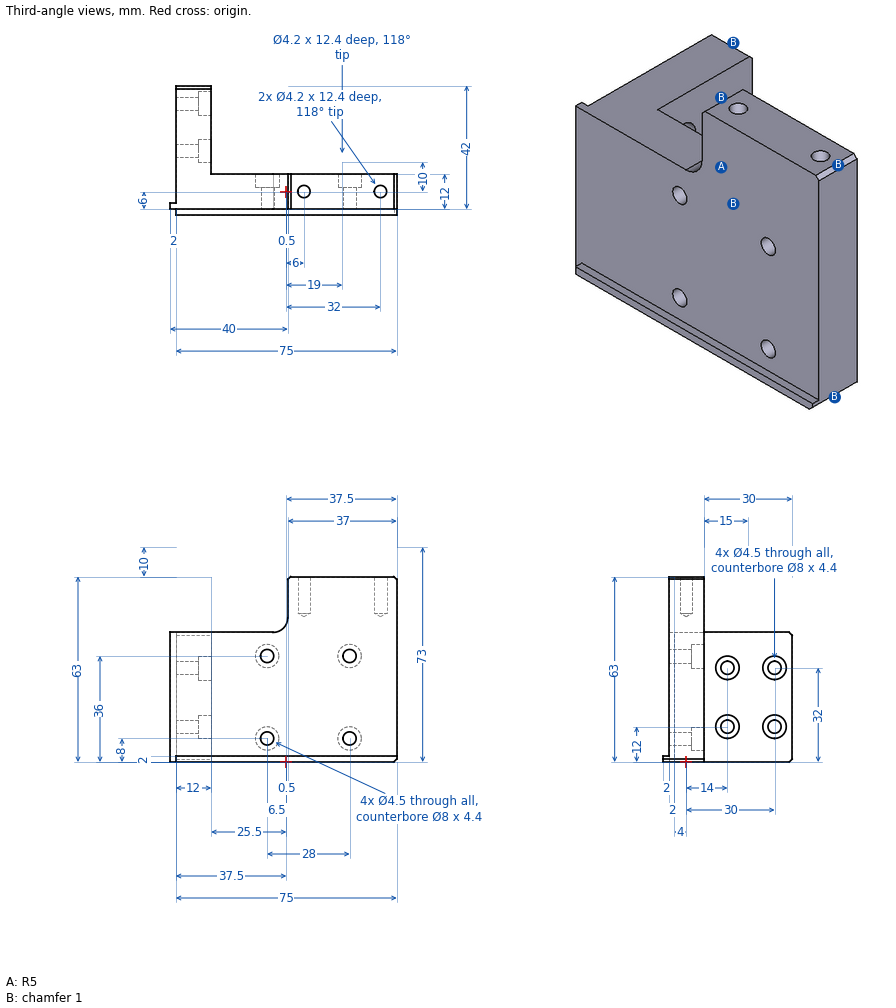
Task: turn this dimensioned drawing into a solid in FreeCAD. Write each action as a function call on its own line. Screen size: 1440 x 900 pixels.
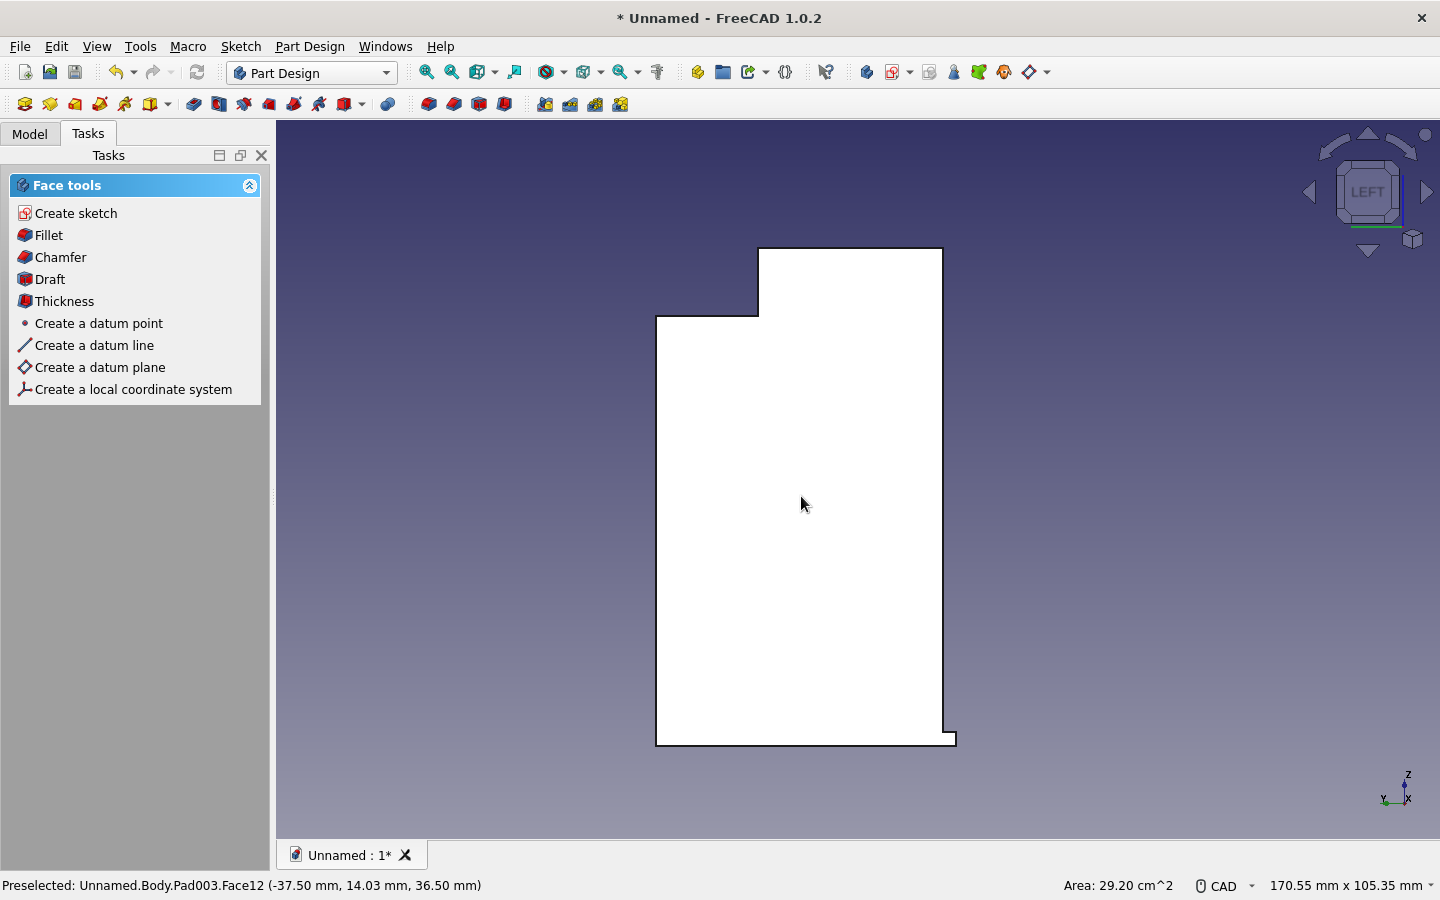
click(892, 72)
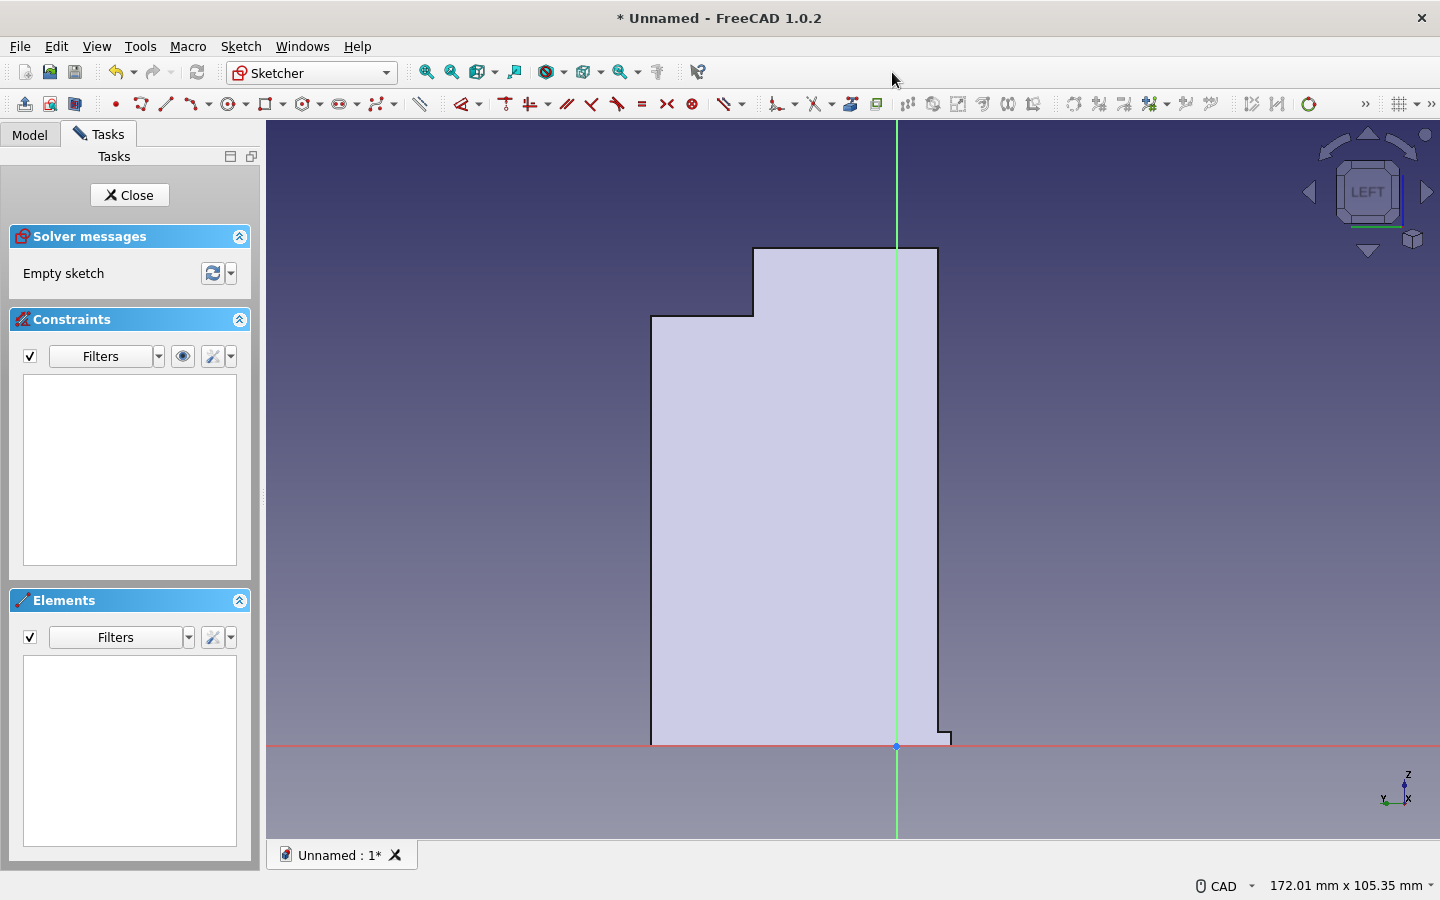
key(g)
key(r)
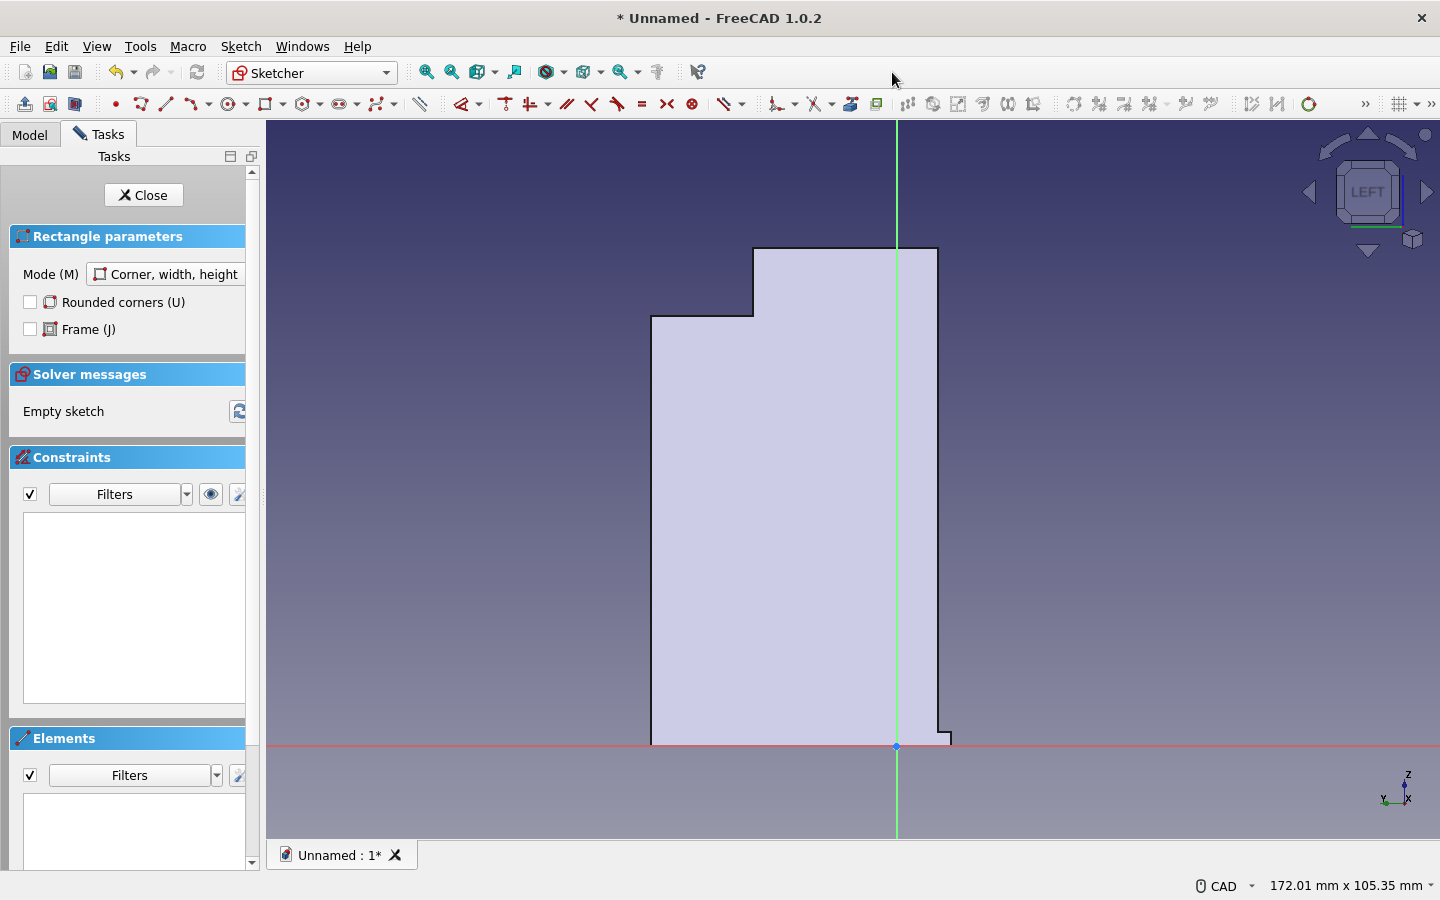
click(924, 316)
click(938, 746)
key(Escape)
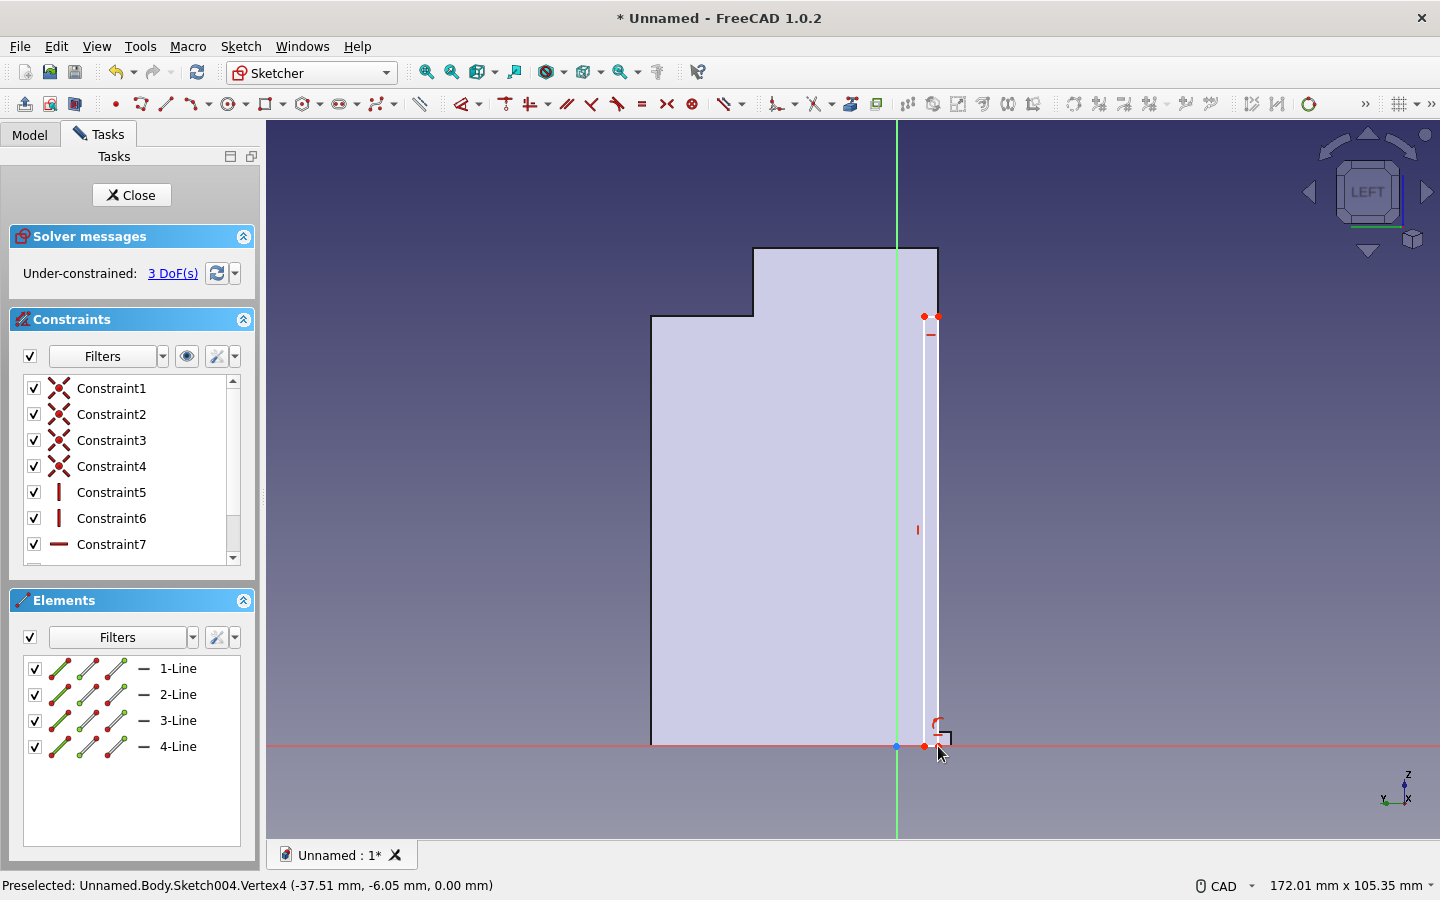
key(d)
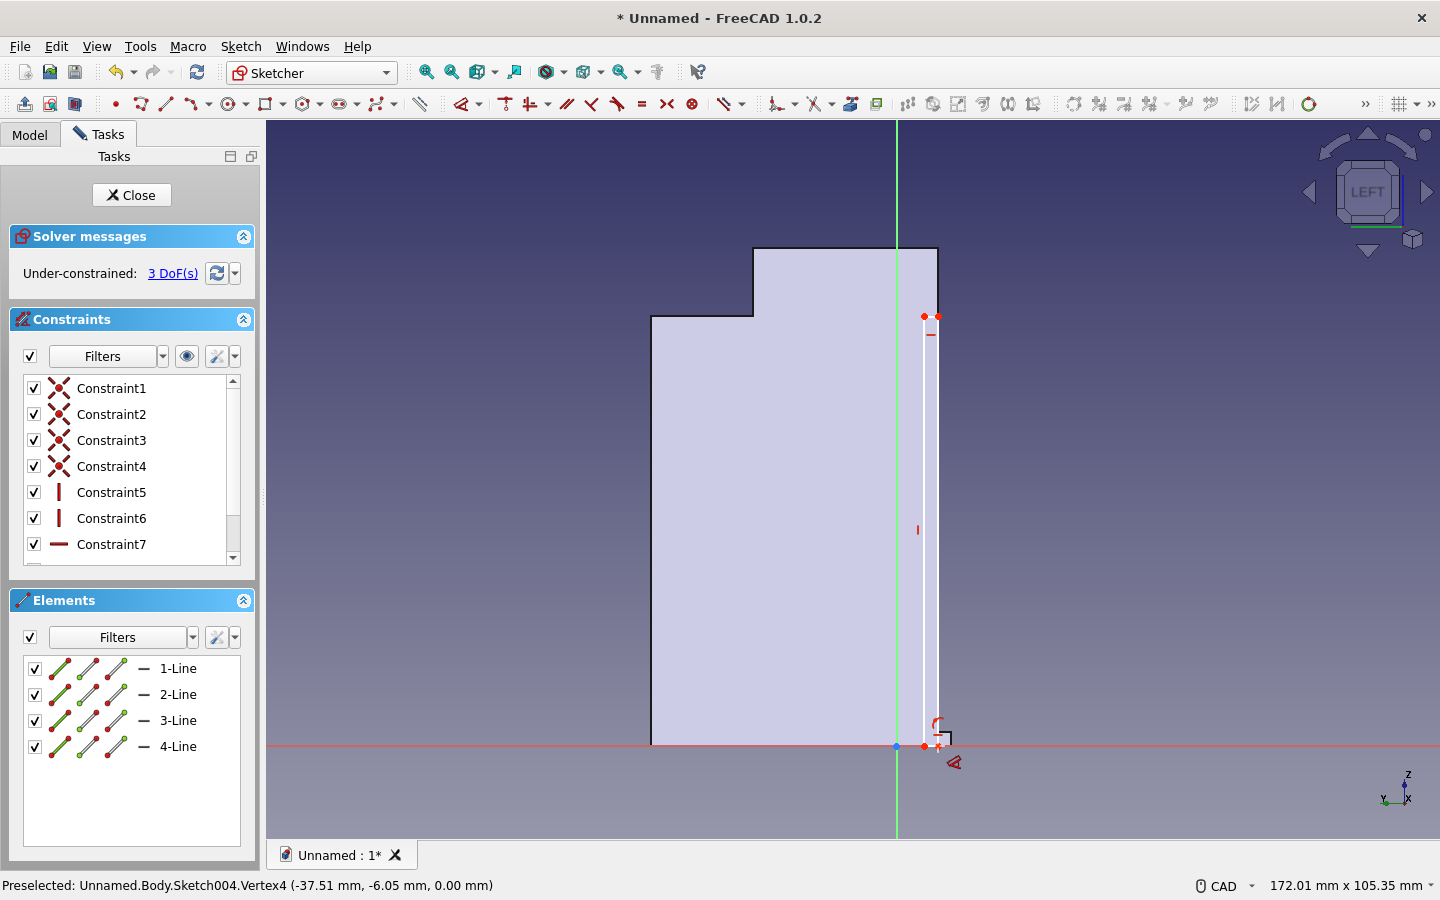
scroll(931, 746, up, 6)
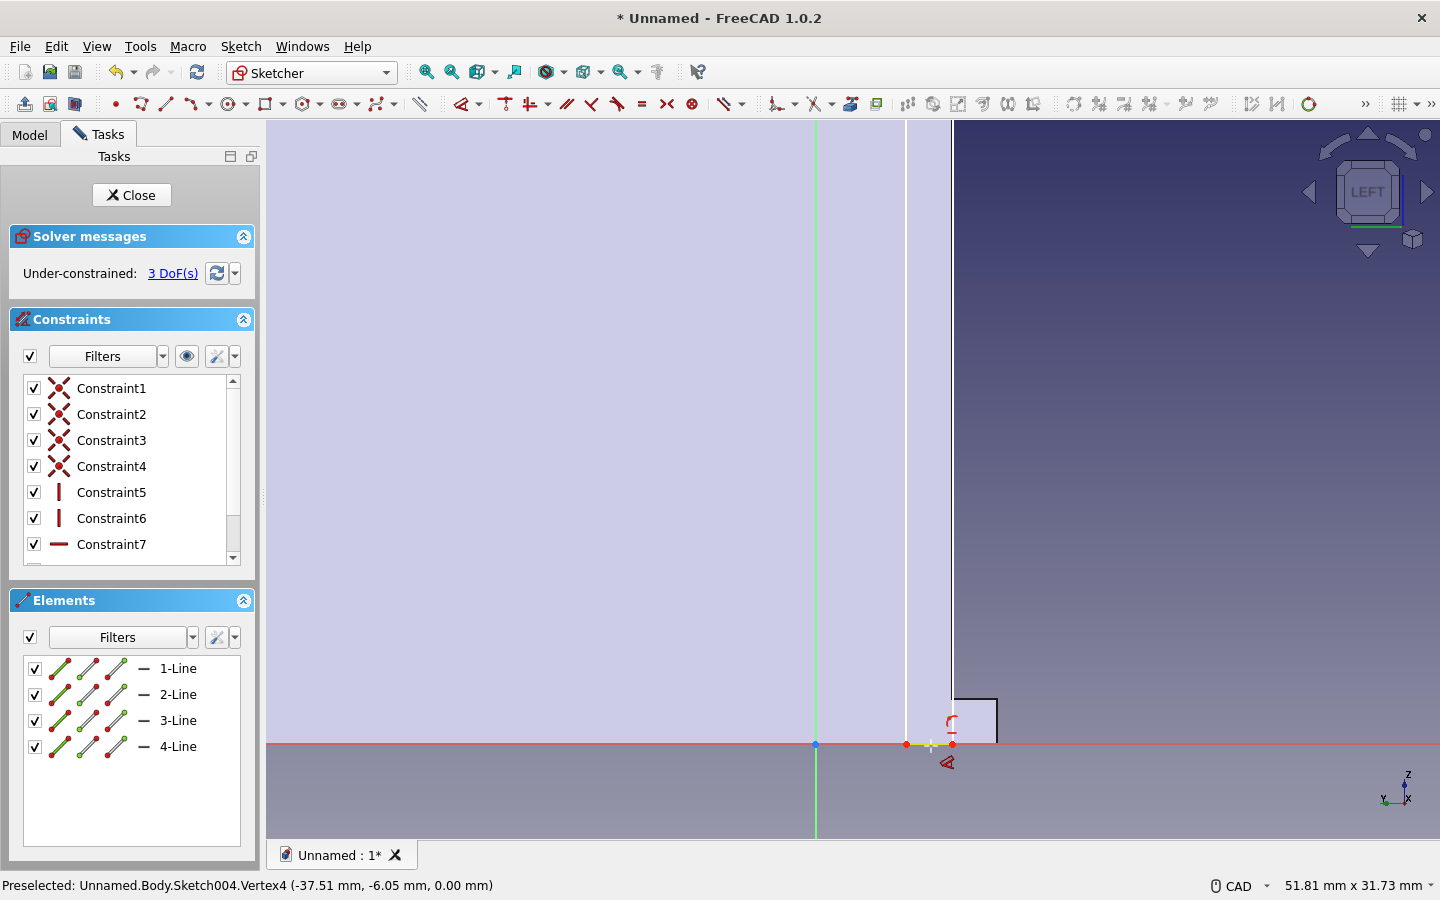
click(930, 744)
click(930, 778)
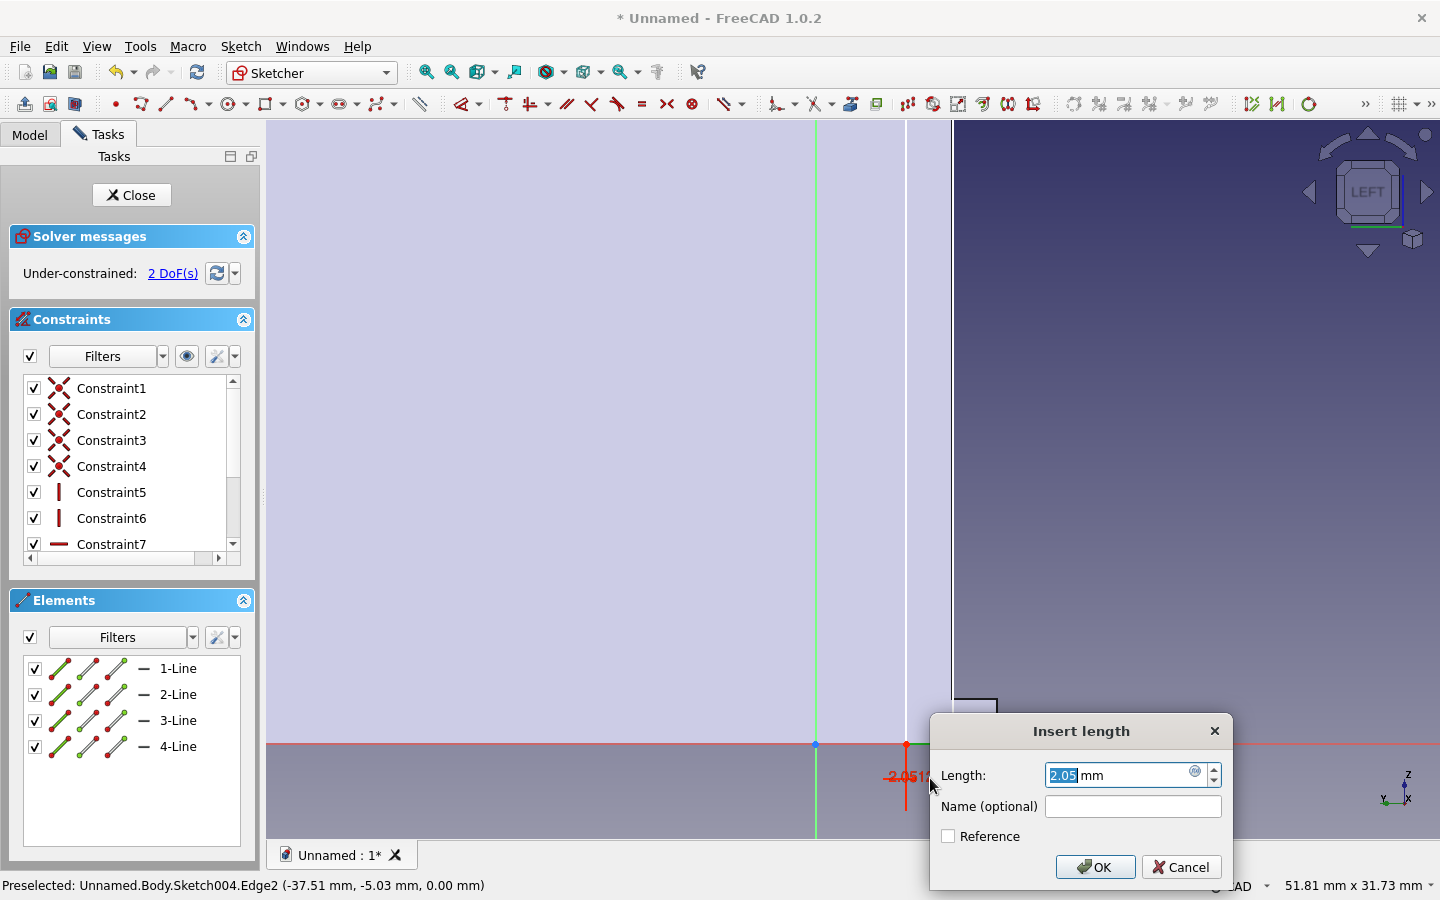
text(2)
key(Return)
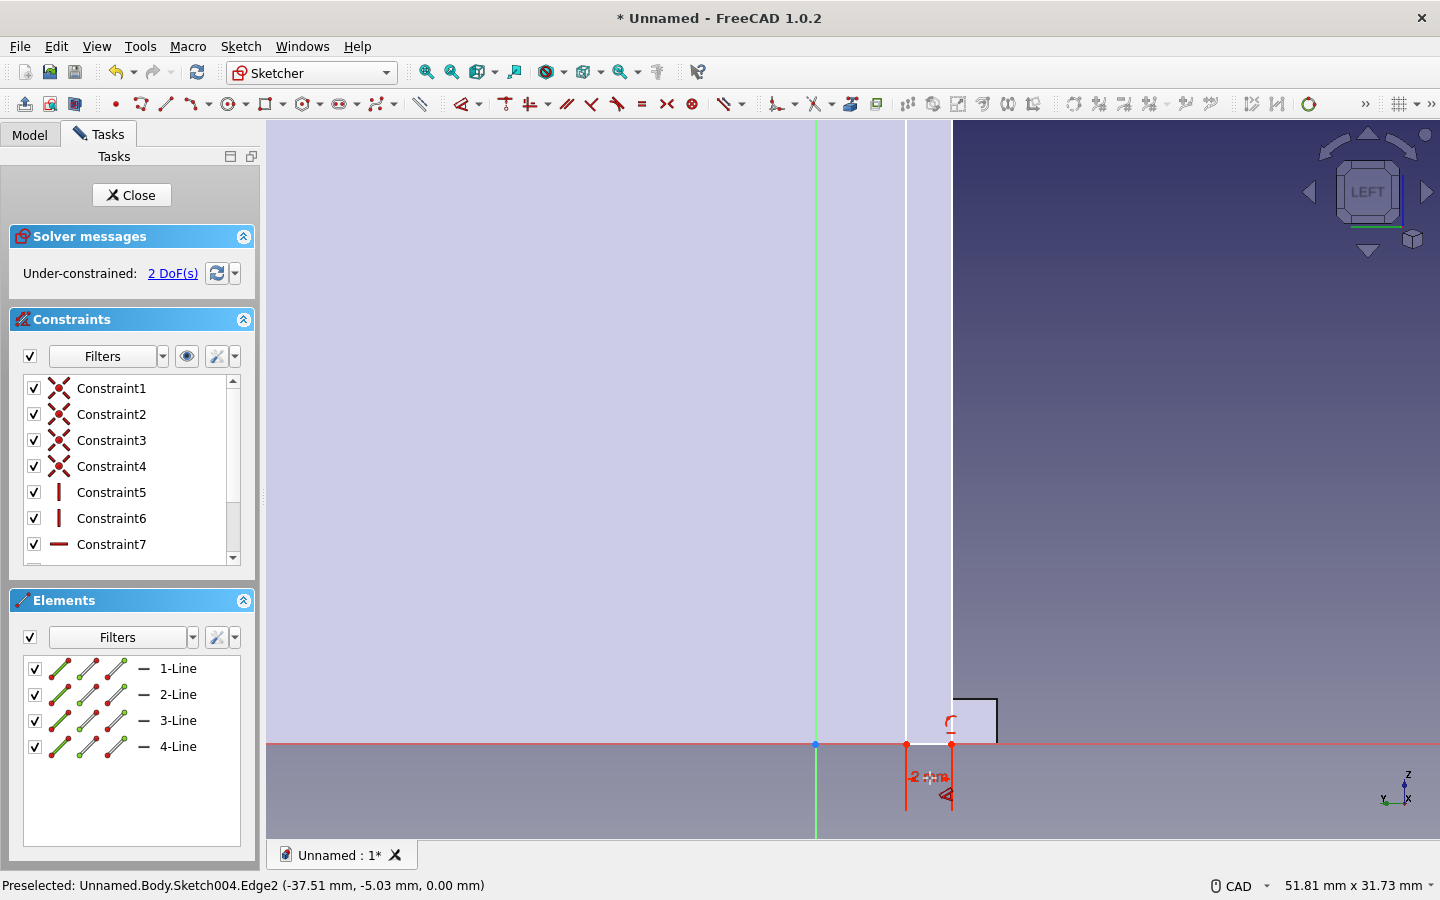
click(906, 317)
click(872, 446)